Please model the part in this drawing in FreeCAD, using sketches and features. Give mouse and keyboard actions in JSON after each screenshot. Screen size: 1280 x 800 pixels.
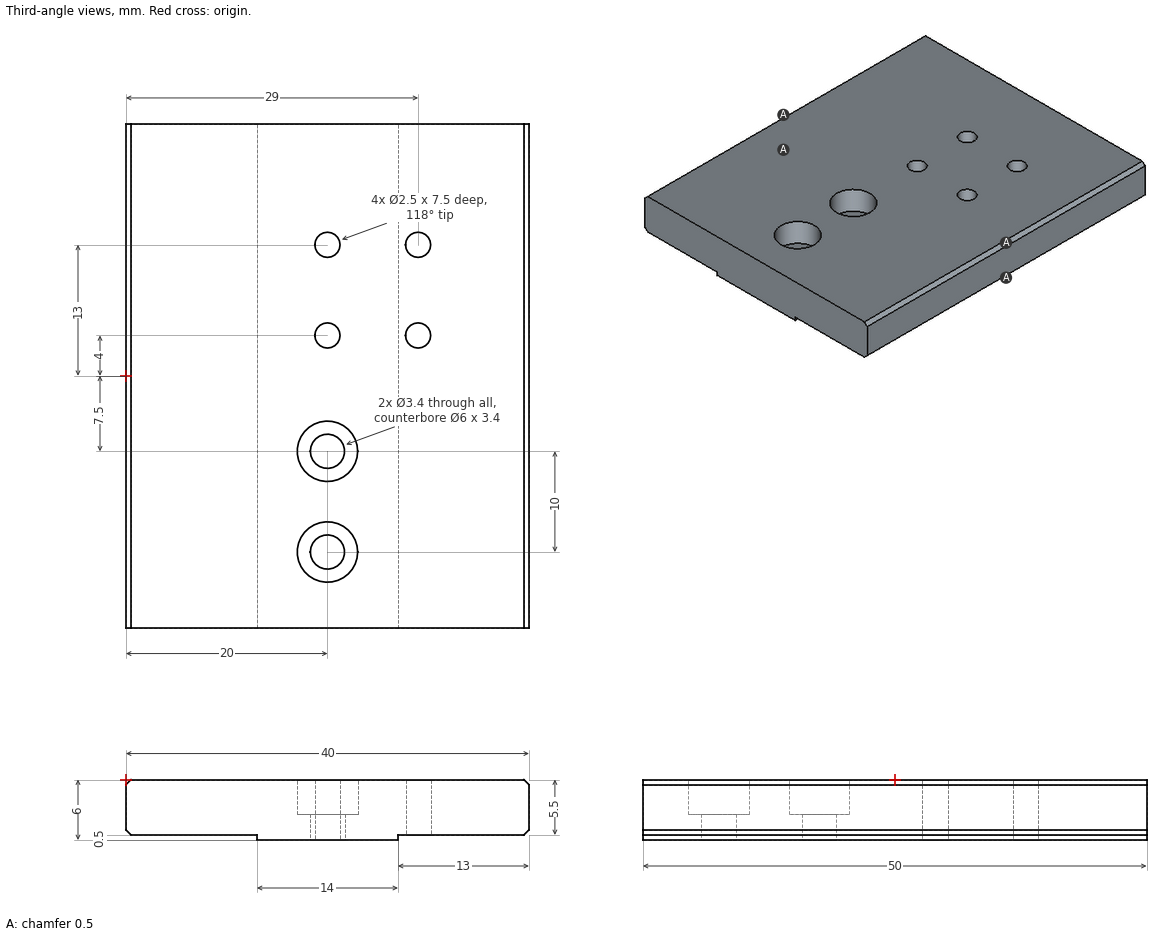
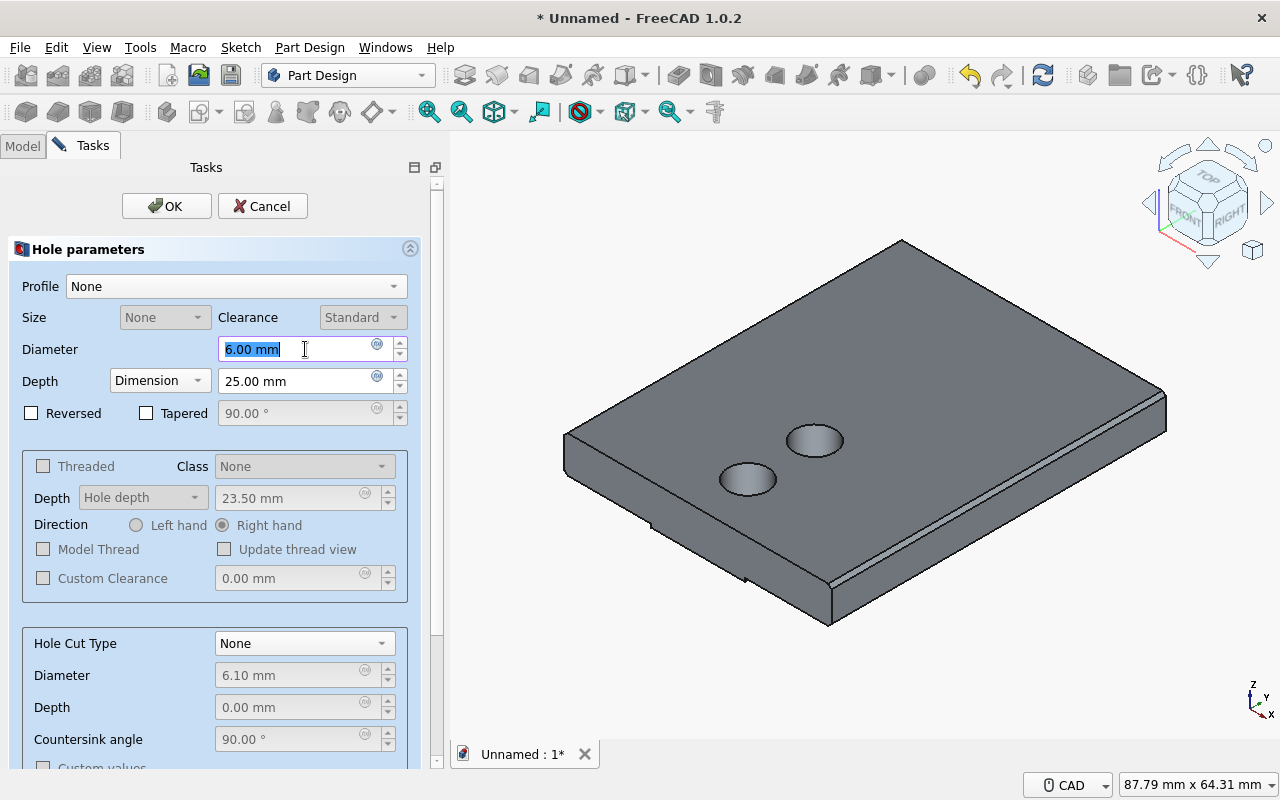
{"action": "type", "text": "3.4"}
{"action": "key", "text": "Tab"}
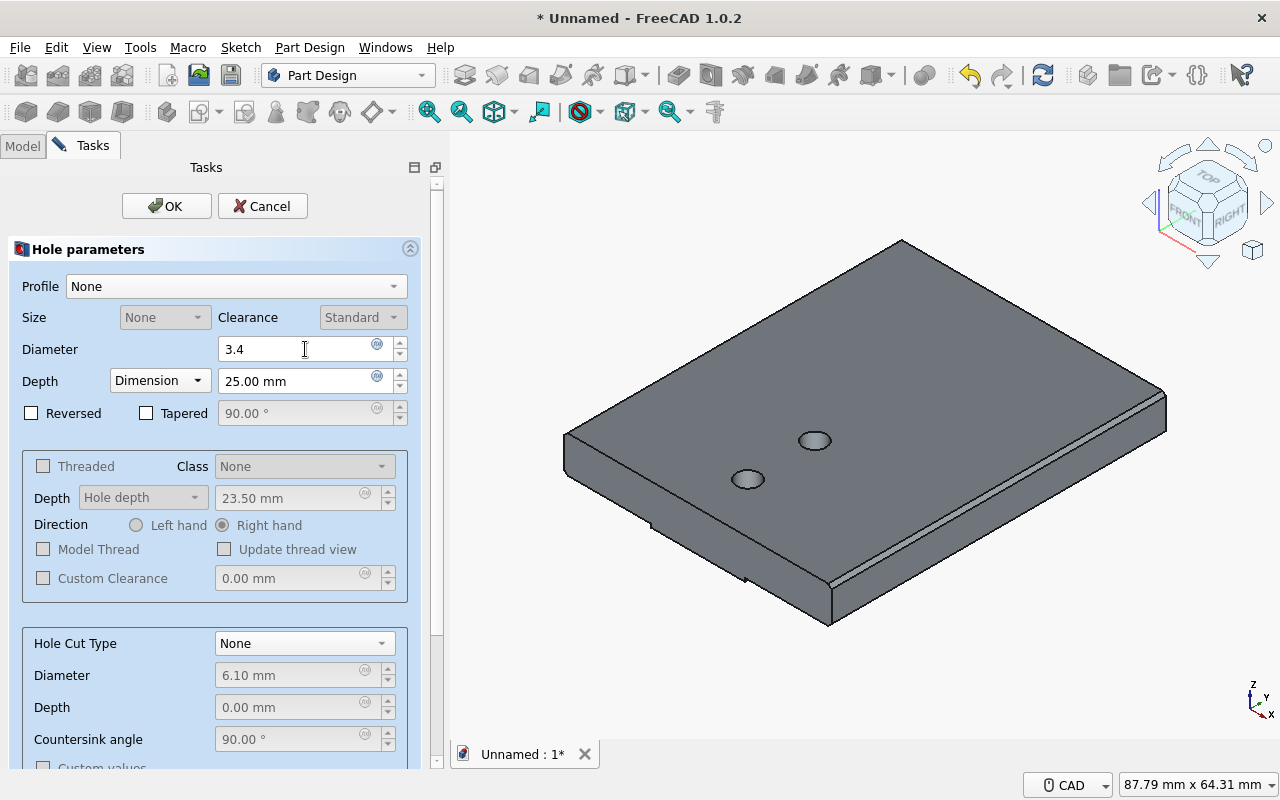
{"action": "left_click", "coordinate": [161, 380]}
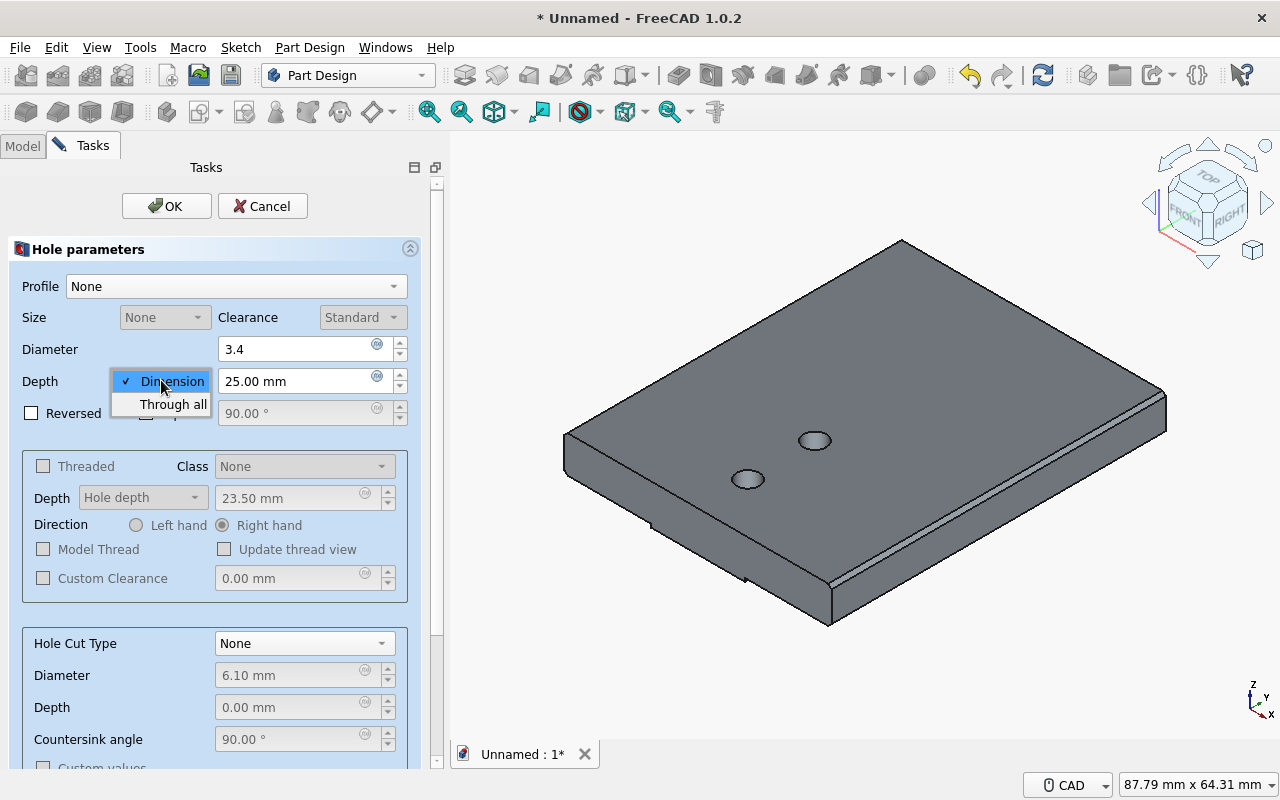
{"action": "left_click", "coordinate": [160, 404]}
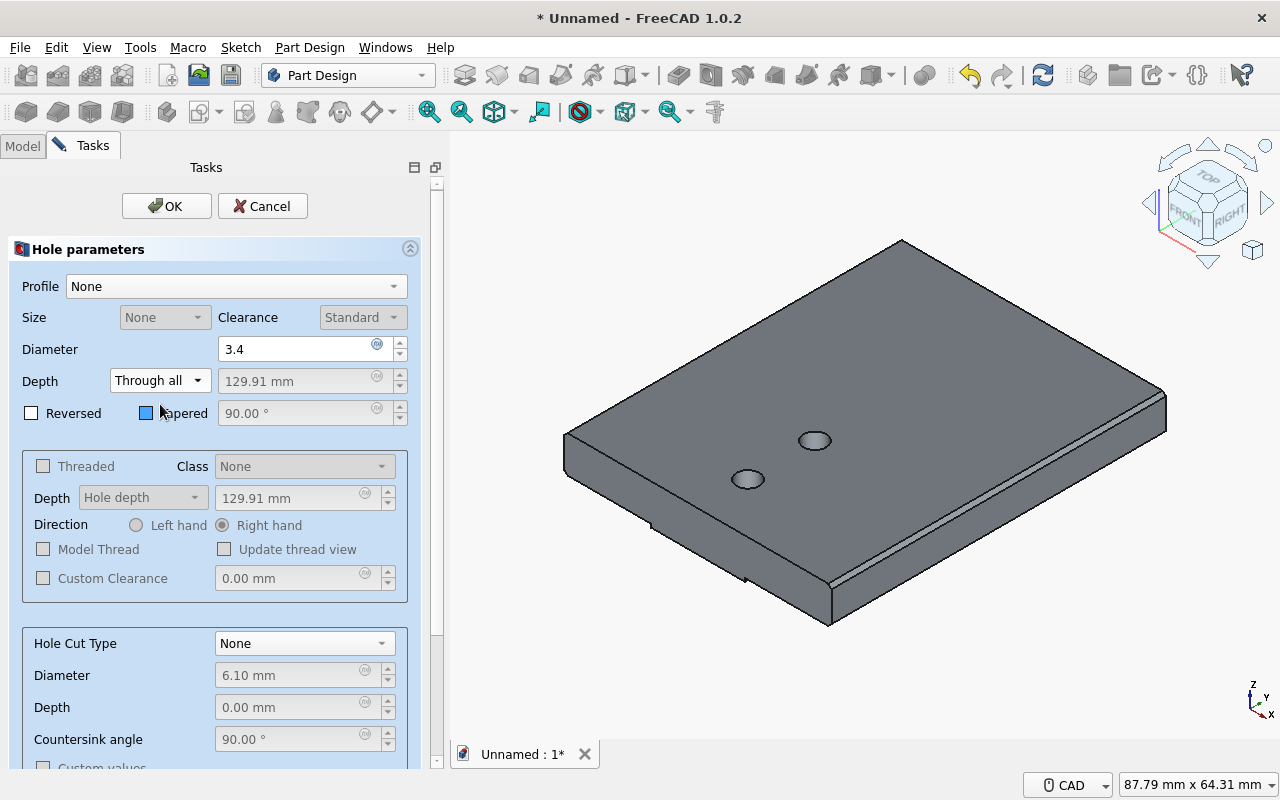
{"action": "left_click", "coordinate": [306, 644]}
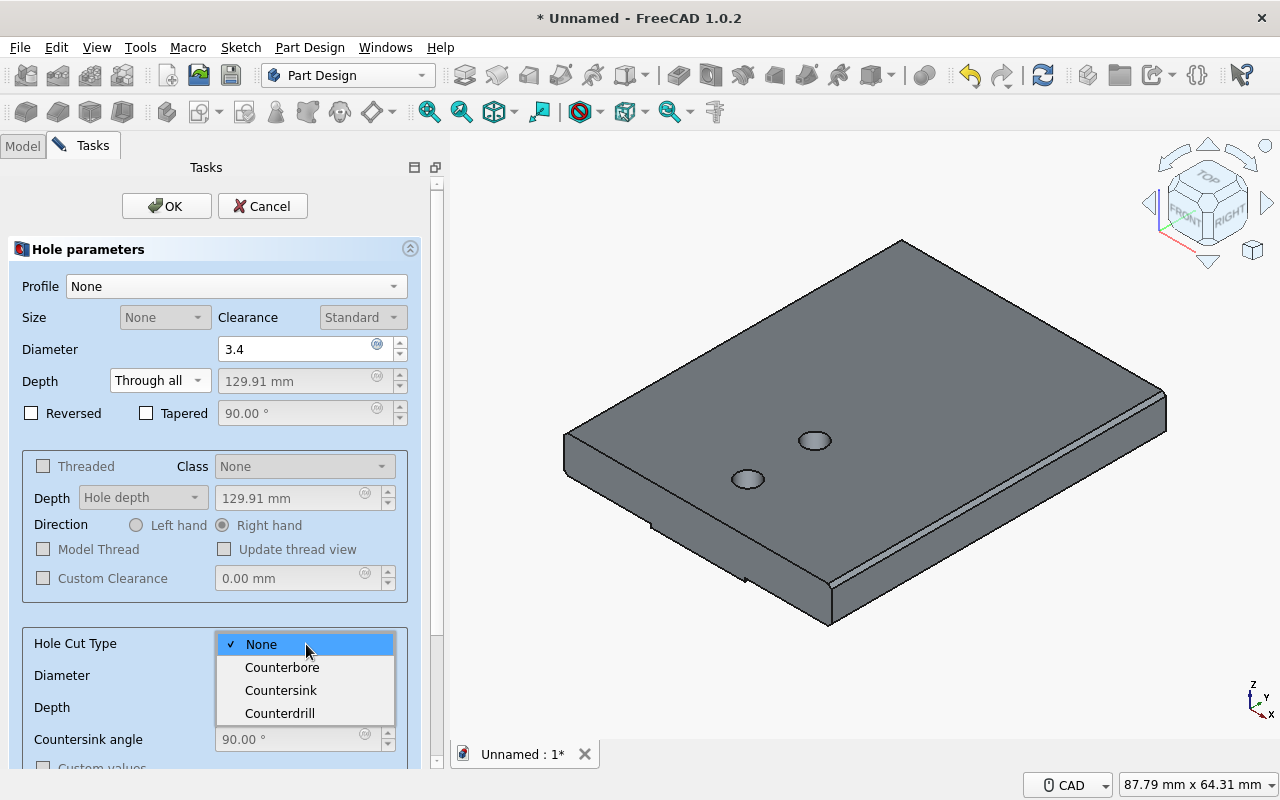
{"action": "left_click", "coordinate": [304, 668]}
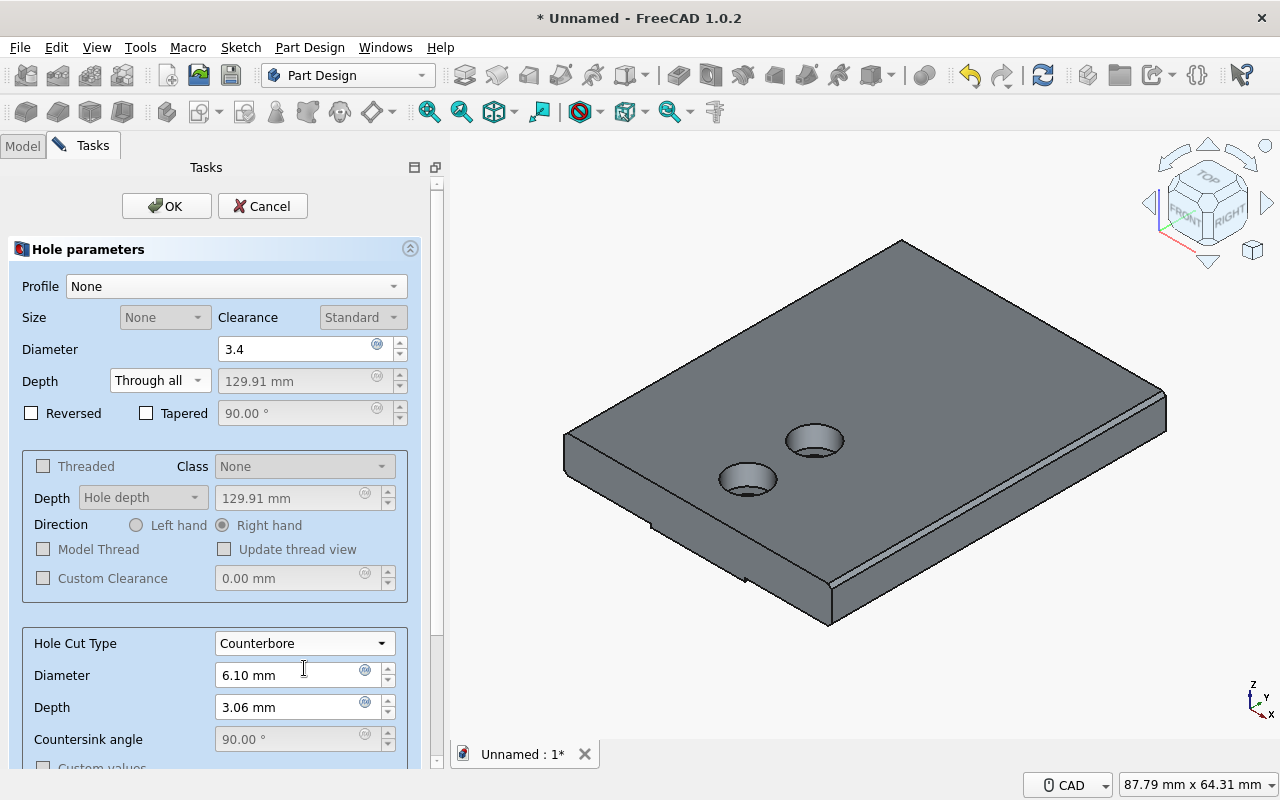
{"action": "triple_click", "coordinate": [298, 675]}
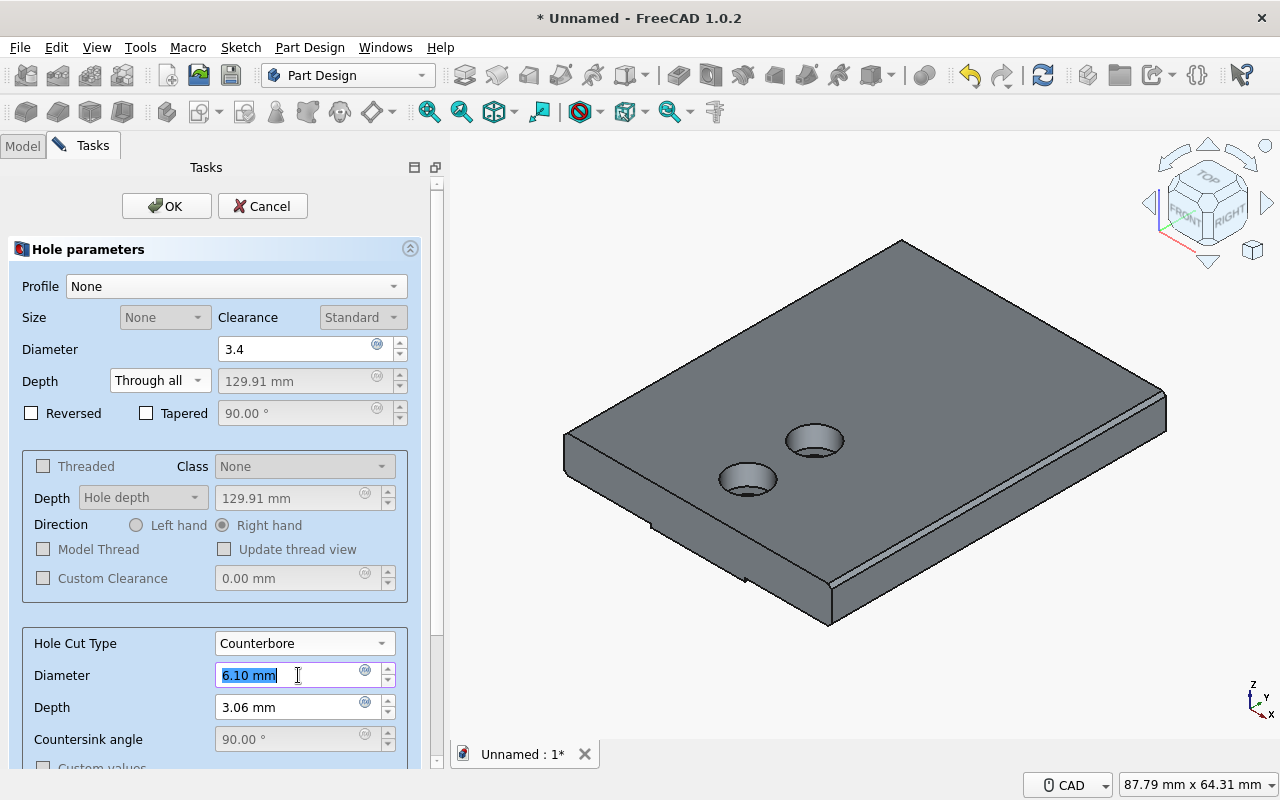
{"action": "type", "text": "6"}
{"action": "key", "text": "Tab"}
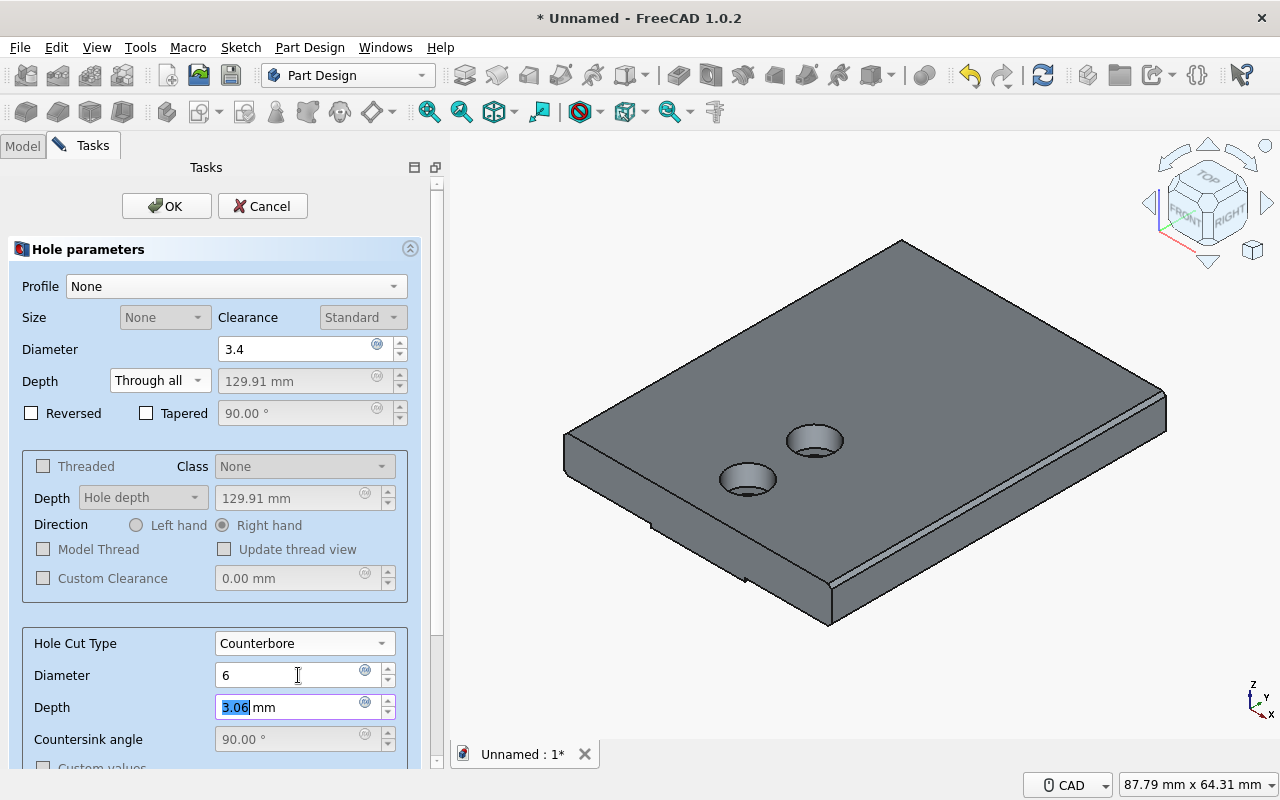
{"action": "type", "text": "3.4"}
{"action": "key", "text": "Tab"}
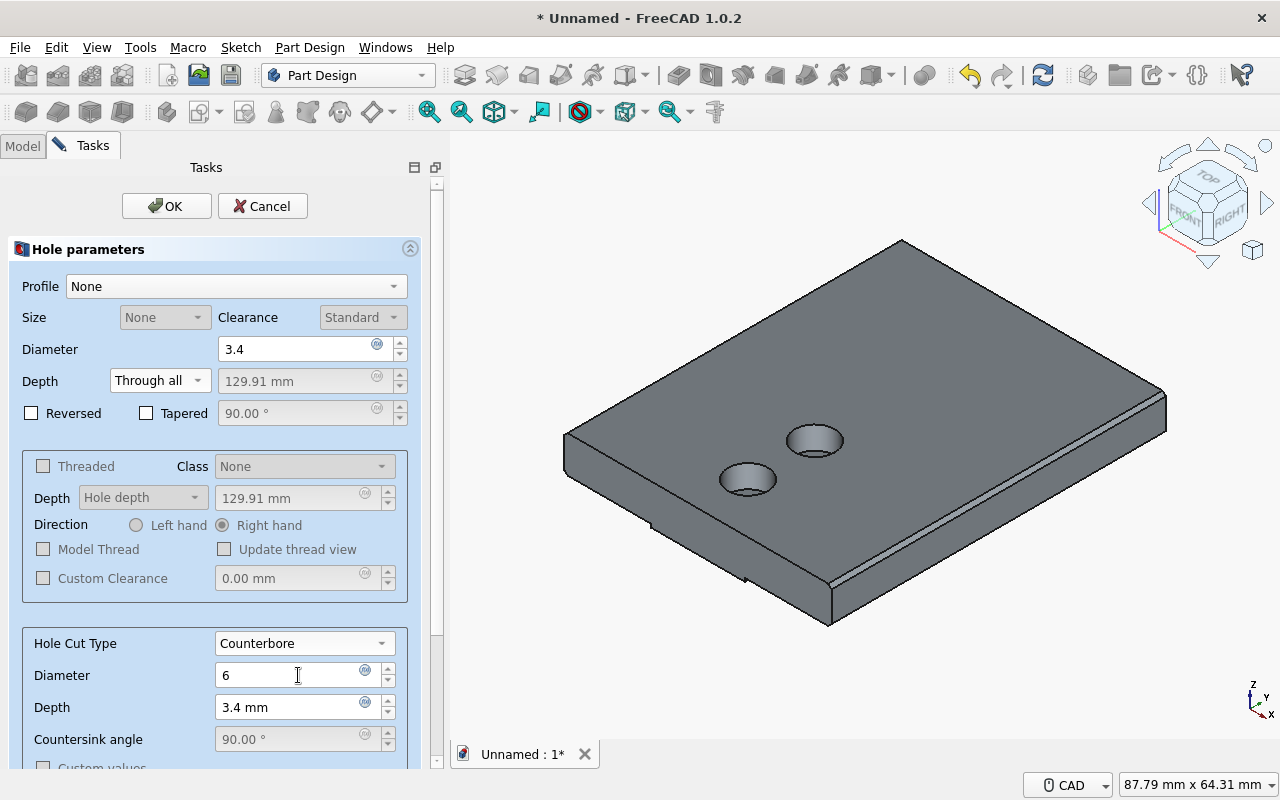
{"action": "left_click", "coordinate": [167, 206]}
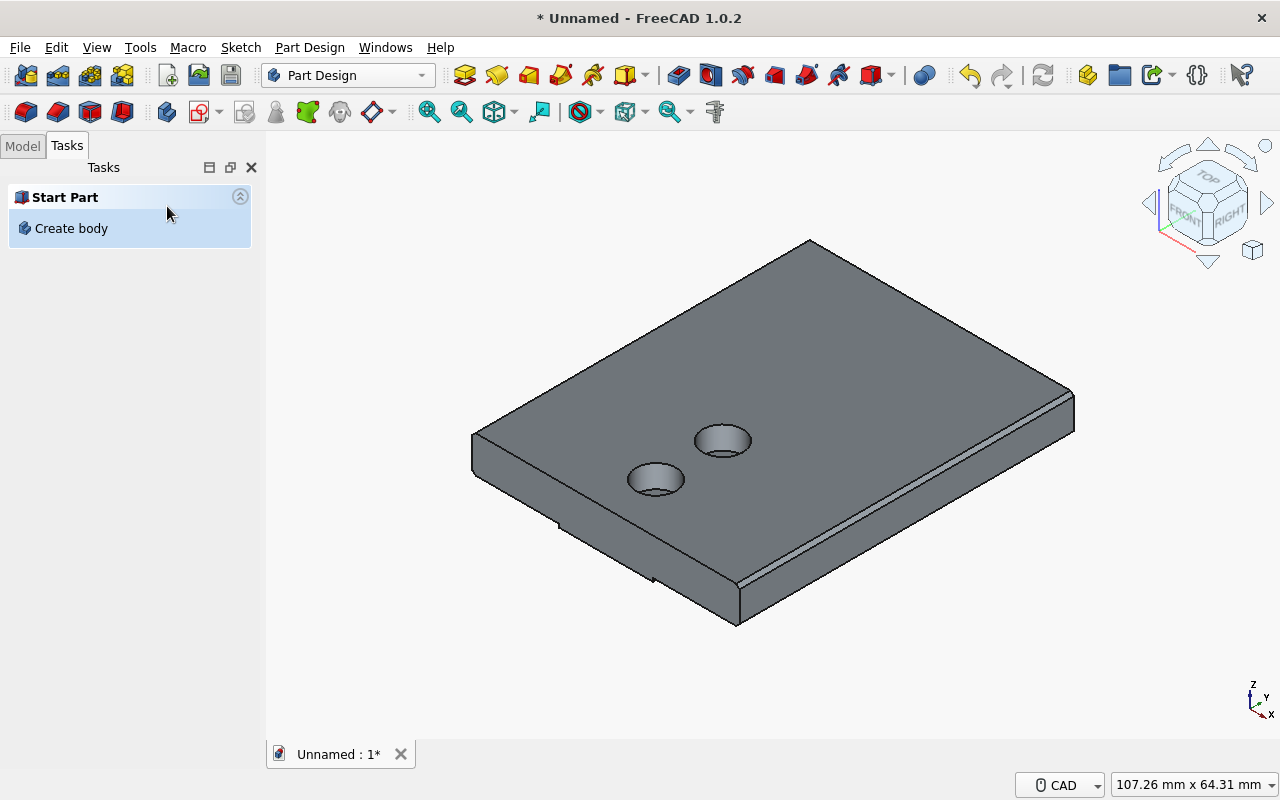
{"action": "left_click", "coordinate": [200, 112]}